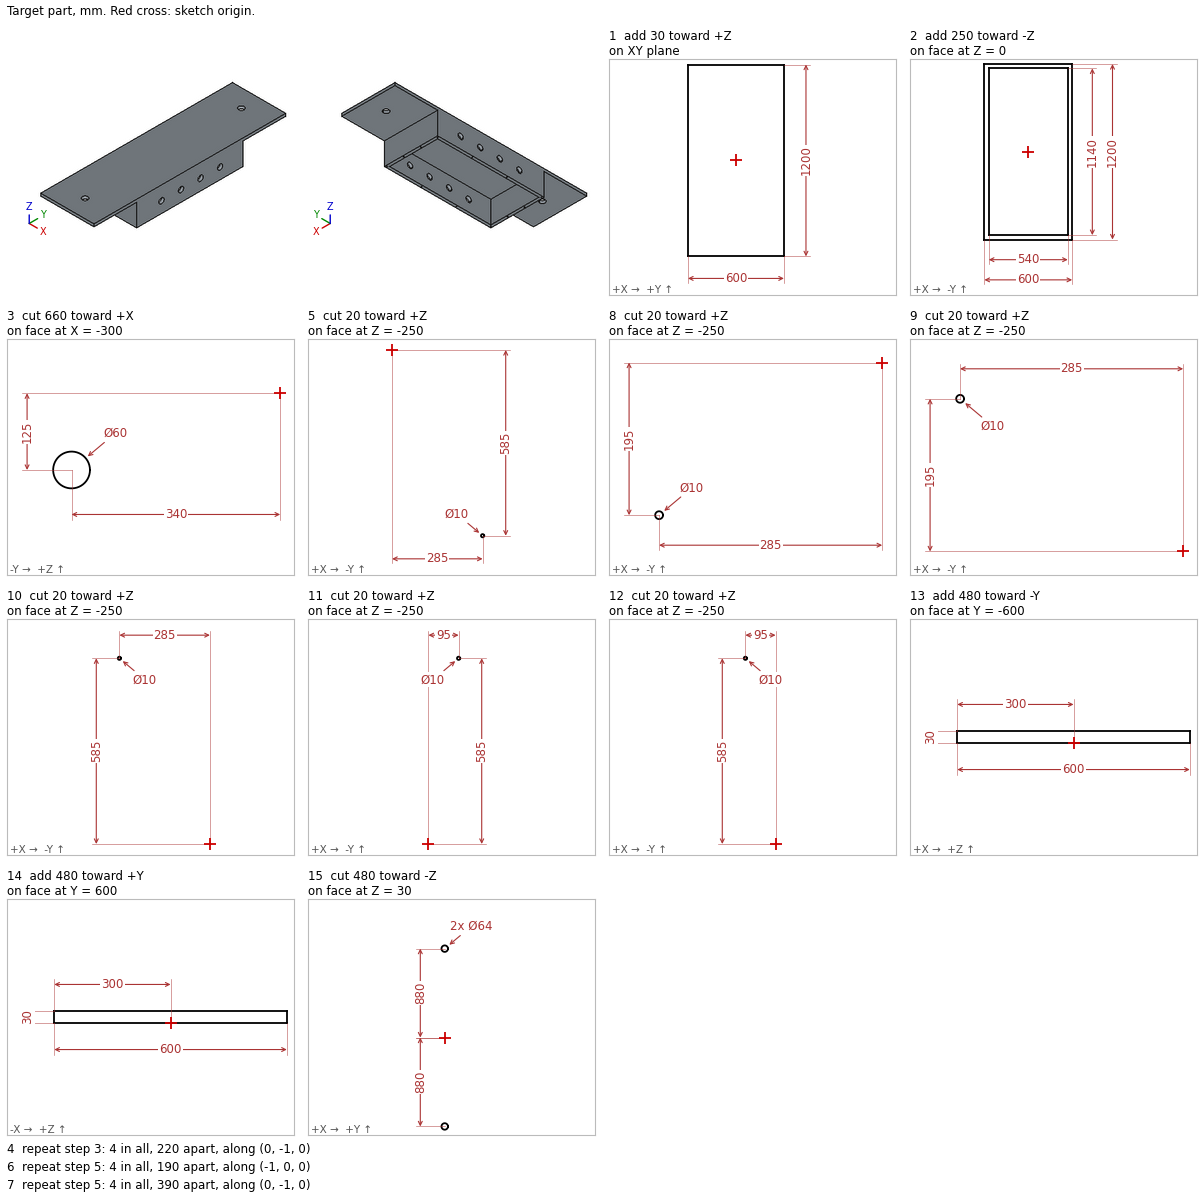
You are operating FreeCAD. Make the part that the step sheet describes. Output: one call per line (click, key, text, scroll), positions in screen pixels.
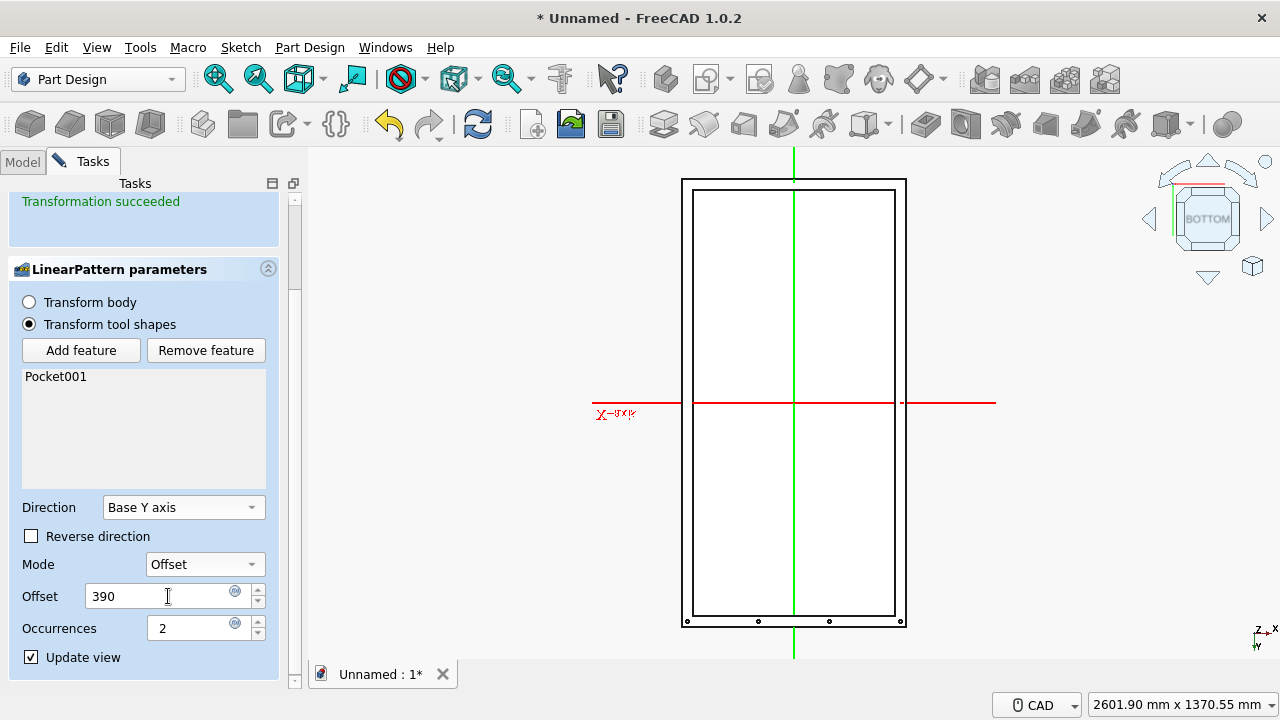
triple_click(198, 628)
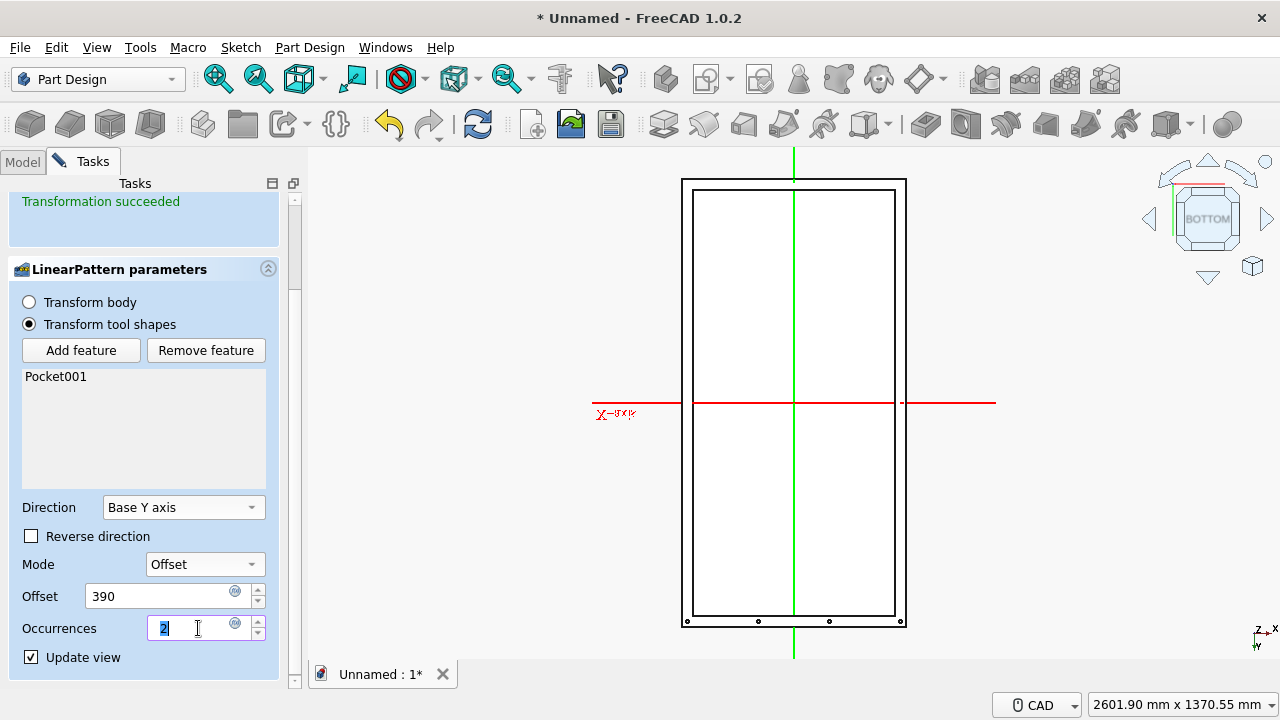
text(4)
key(Tab)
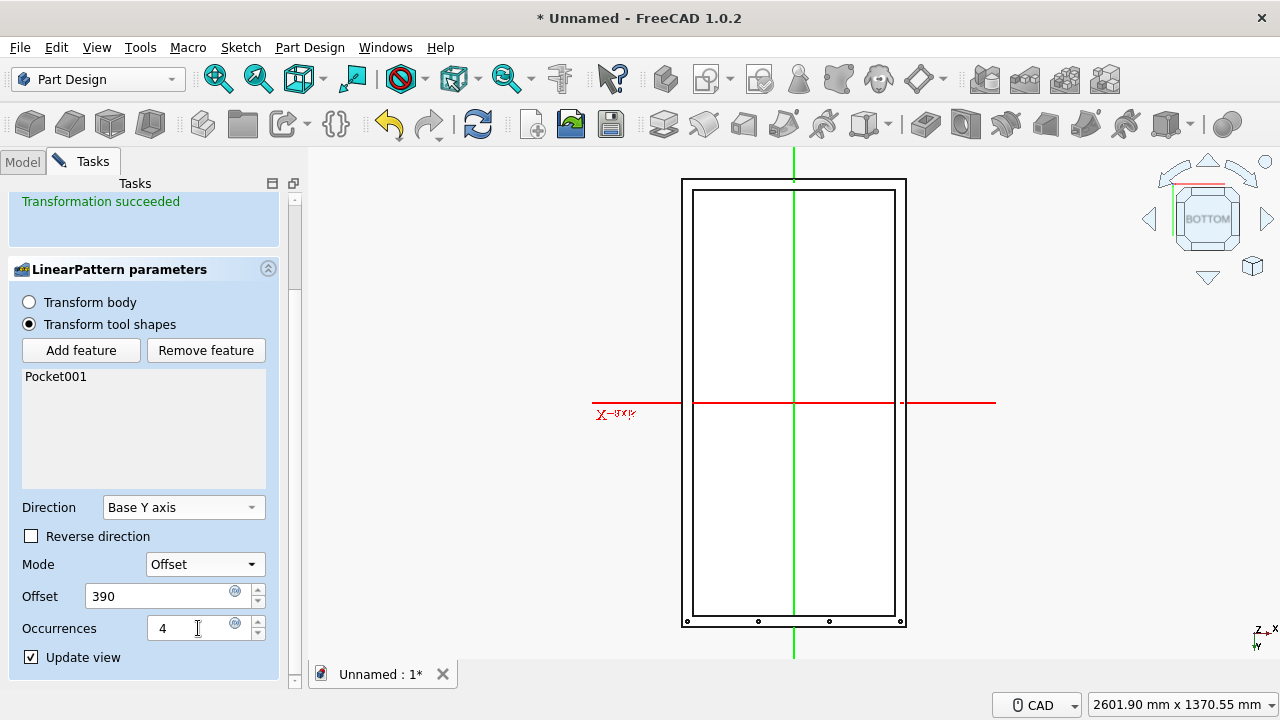
click(30, 536)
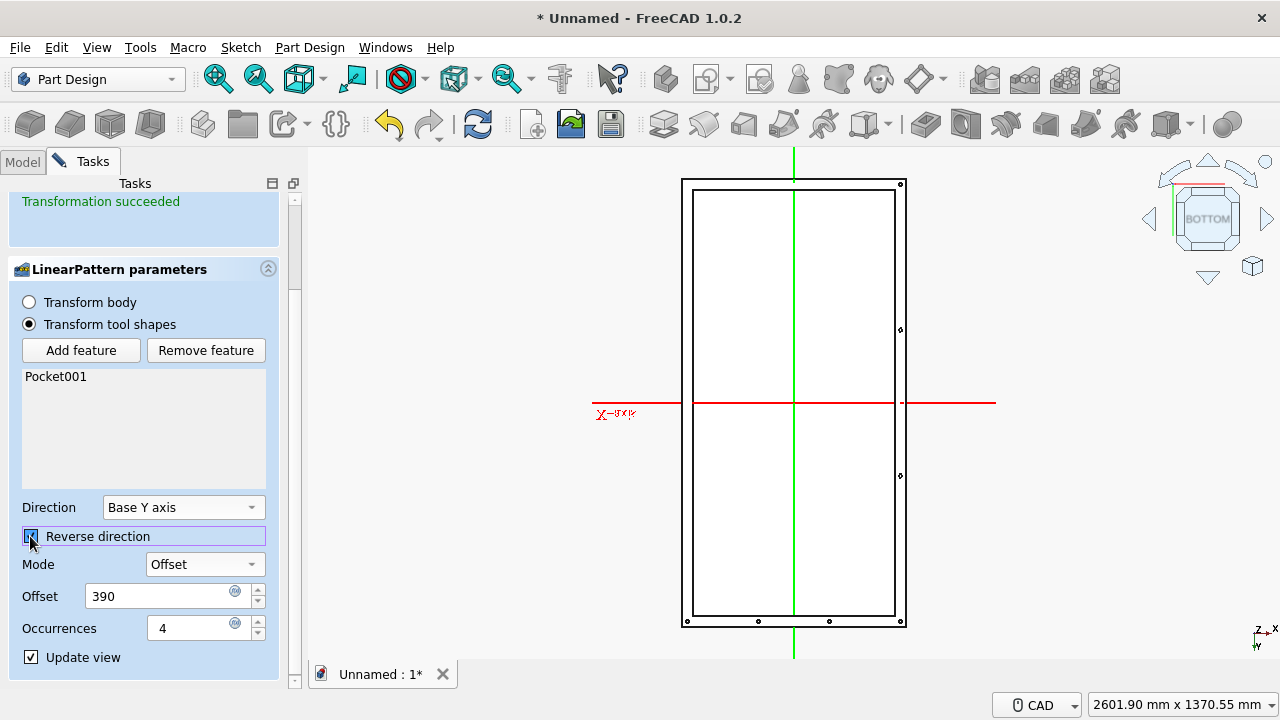
scroll(295, 440, up, 3)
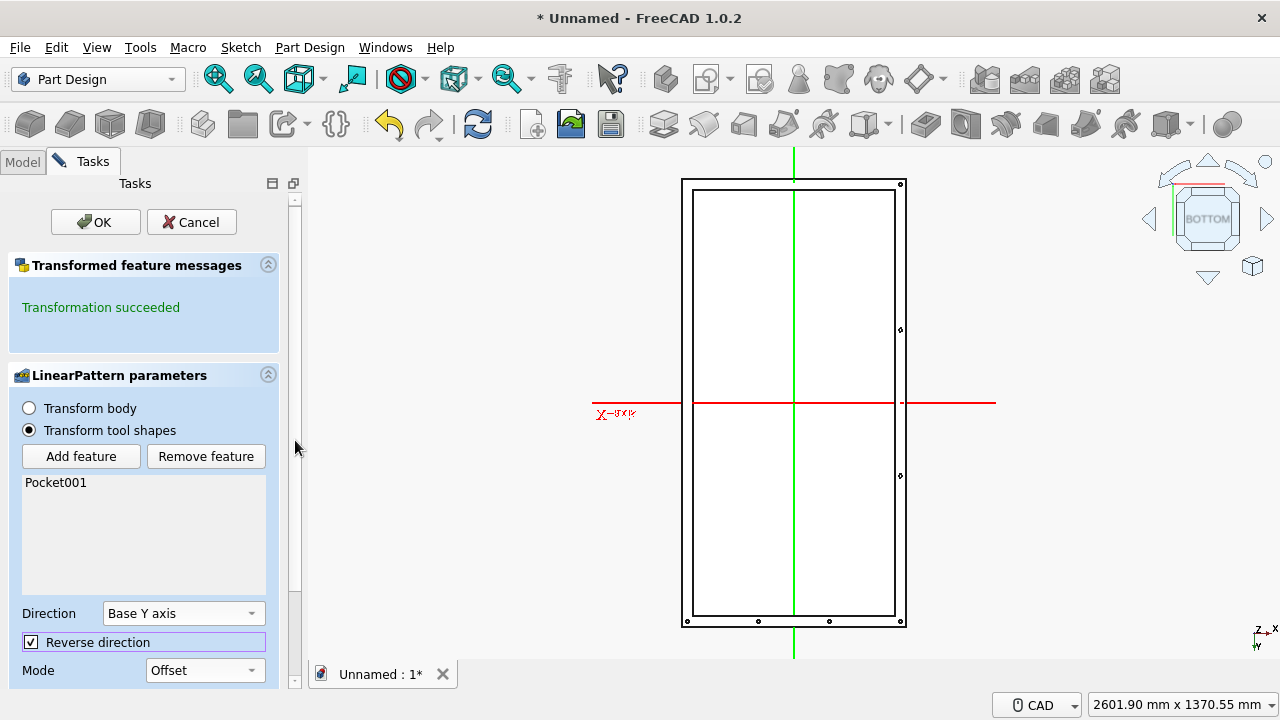
click(96, 222)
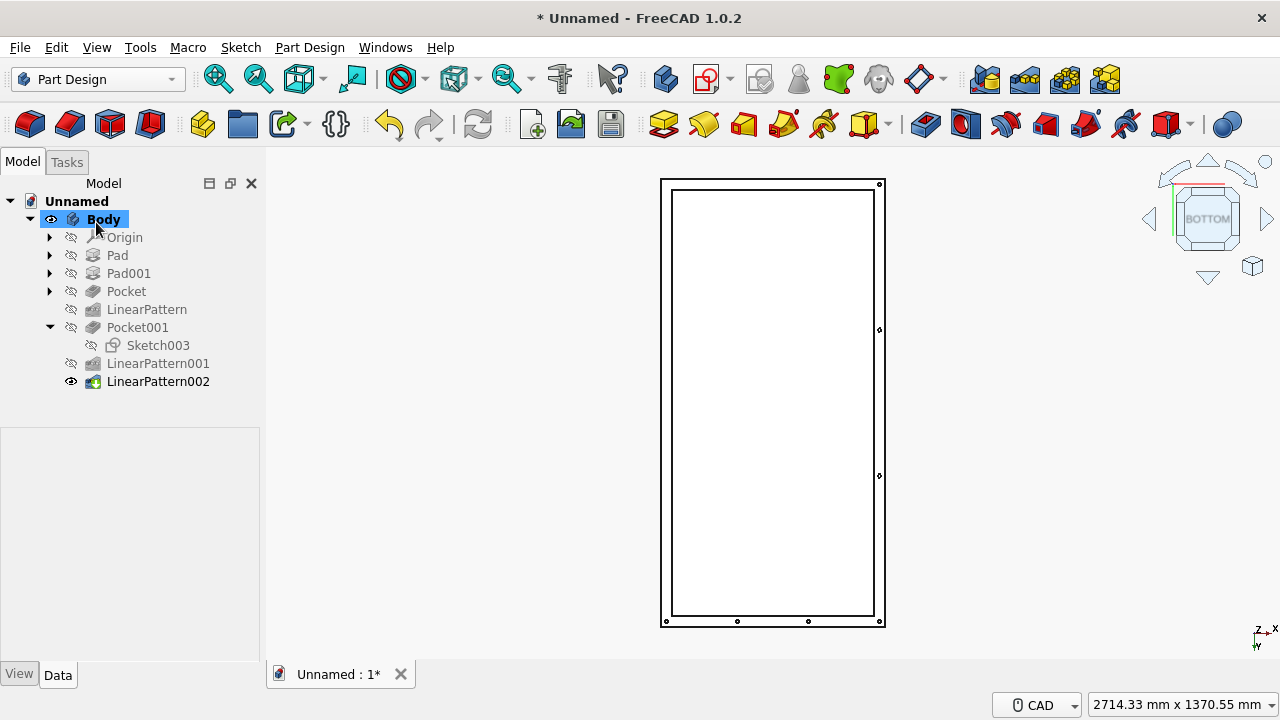
scroll(880, 426, up, 4)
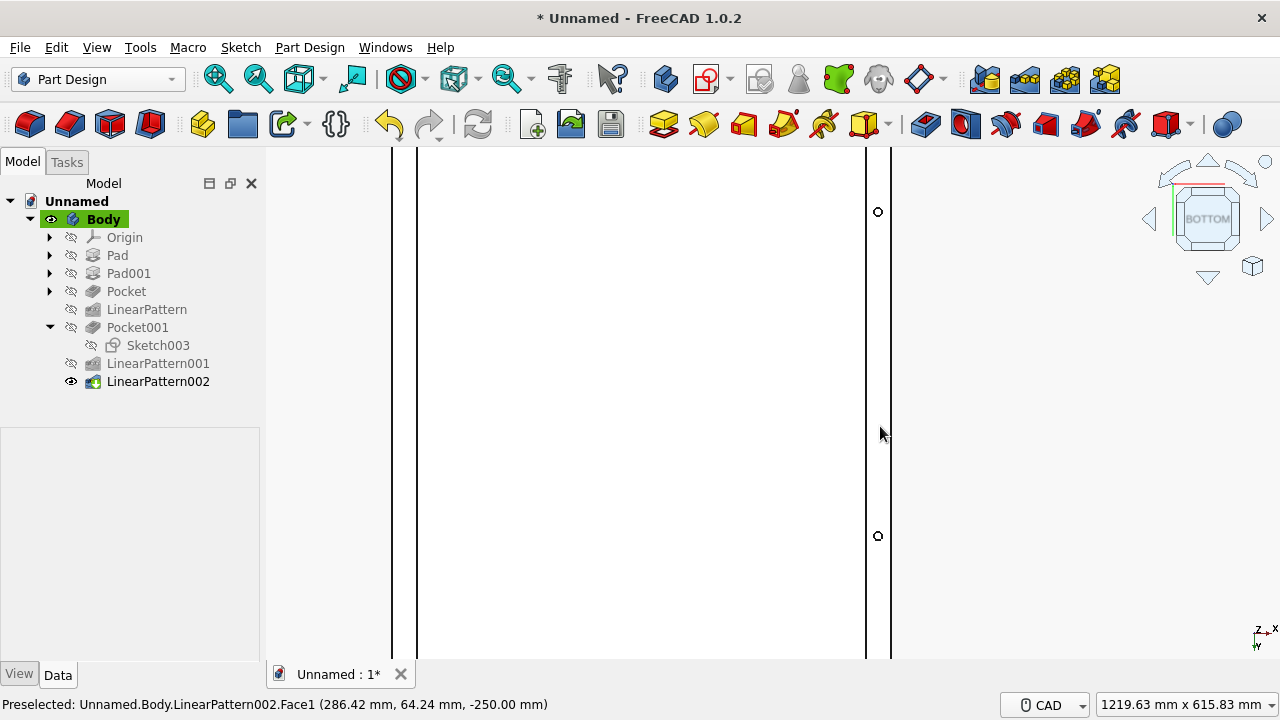
click(878, 426)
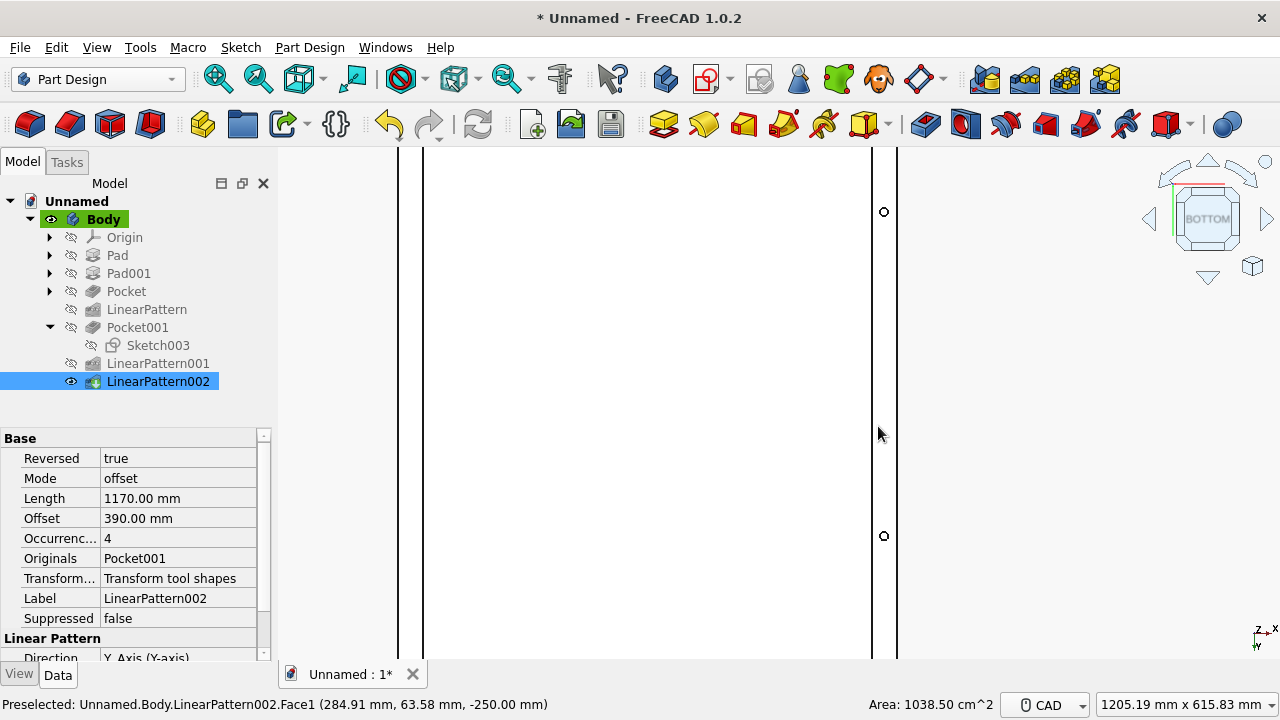
click(706, 80)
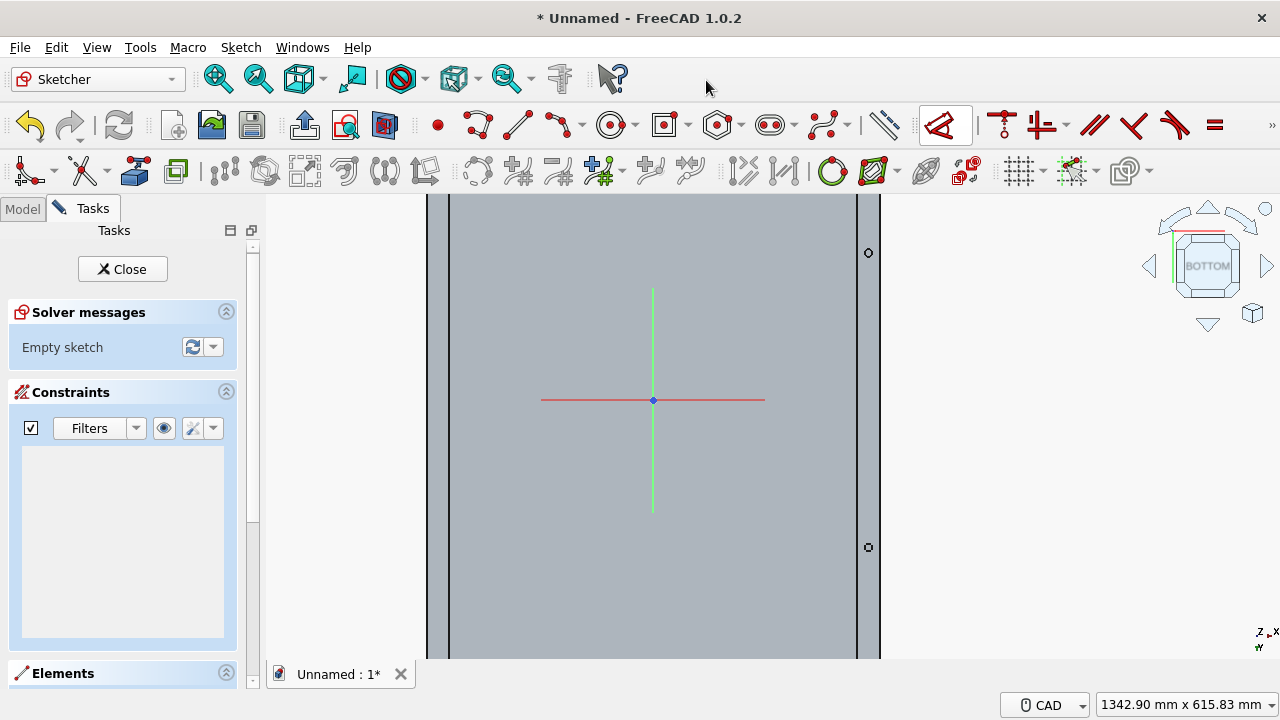
scroll(424, 554, up, 15)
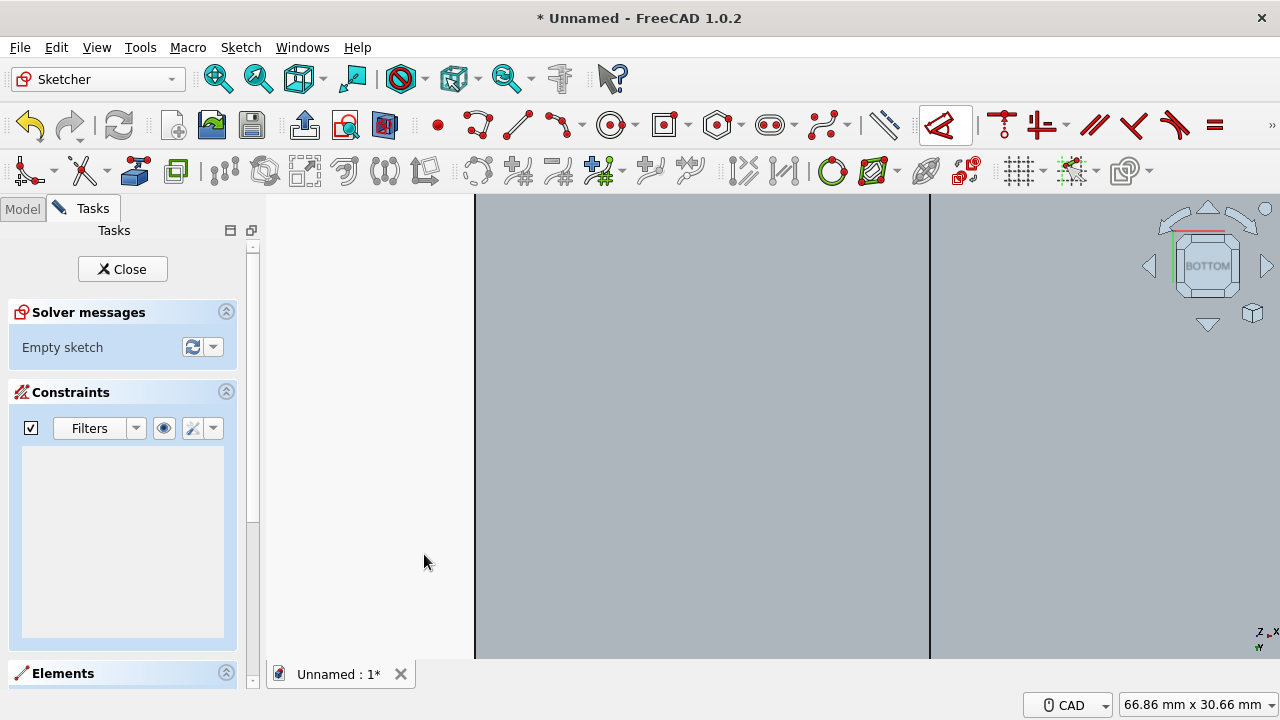
scroll(701, 388, up, 3)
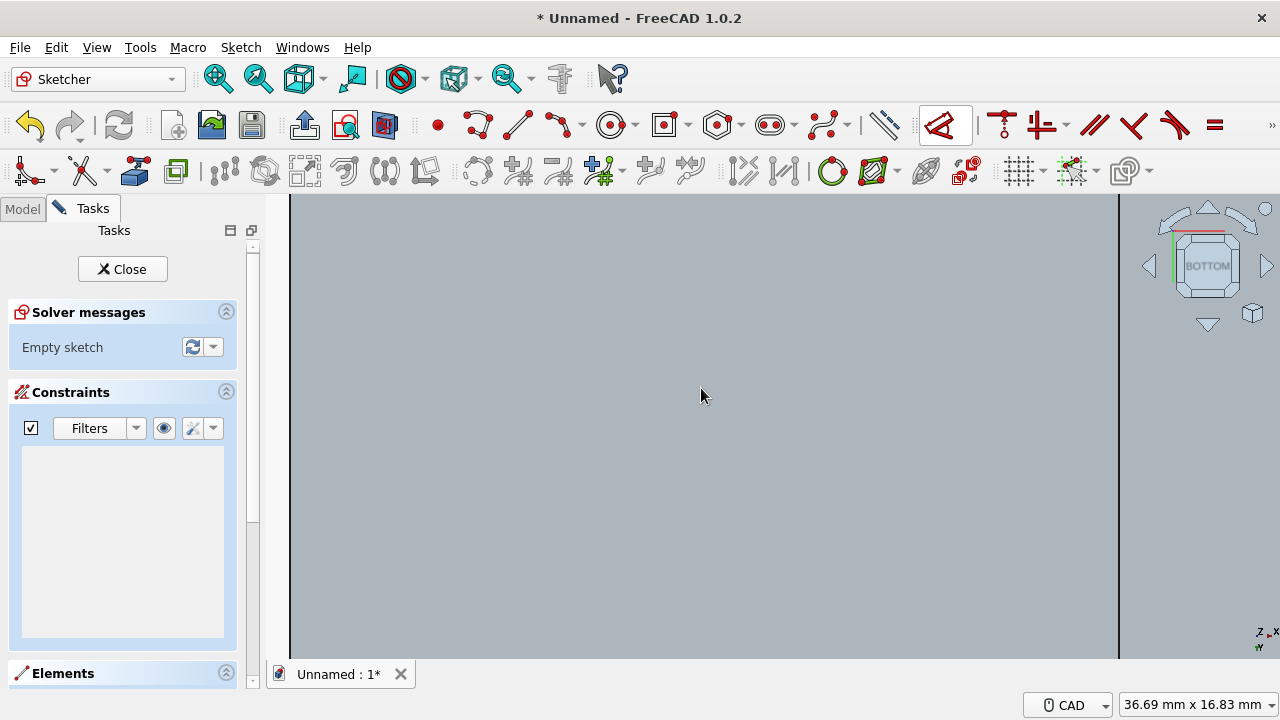
click(612, 126)